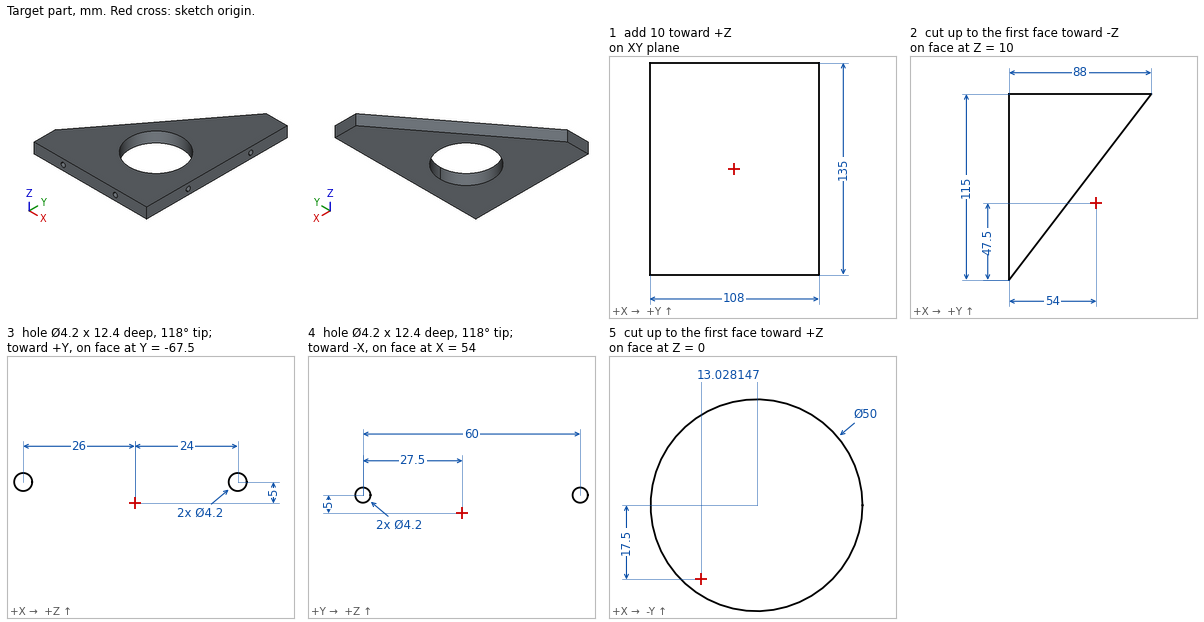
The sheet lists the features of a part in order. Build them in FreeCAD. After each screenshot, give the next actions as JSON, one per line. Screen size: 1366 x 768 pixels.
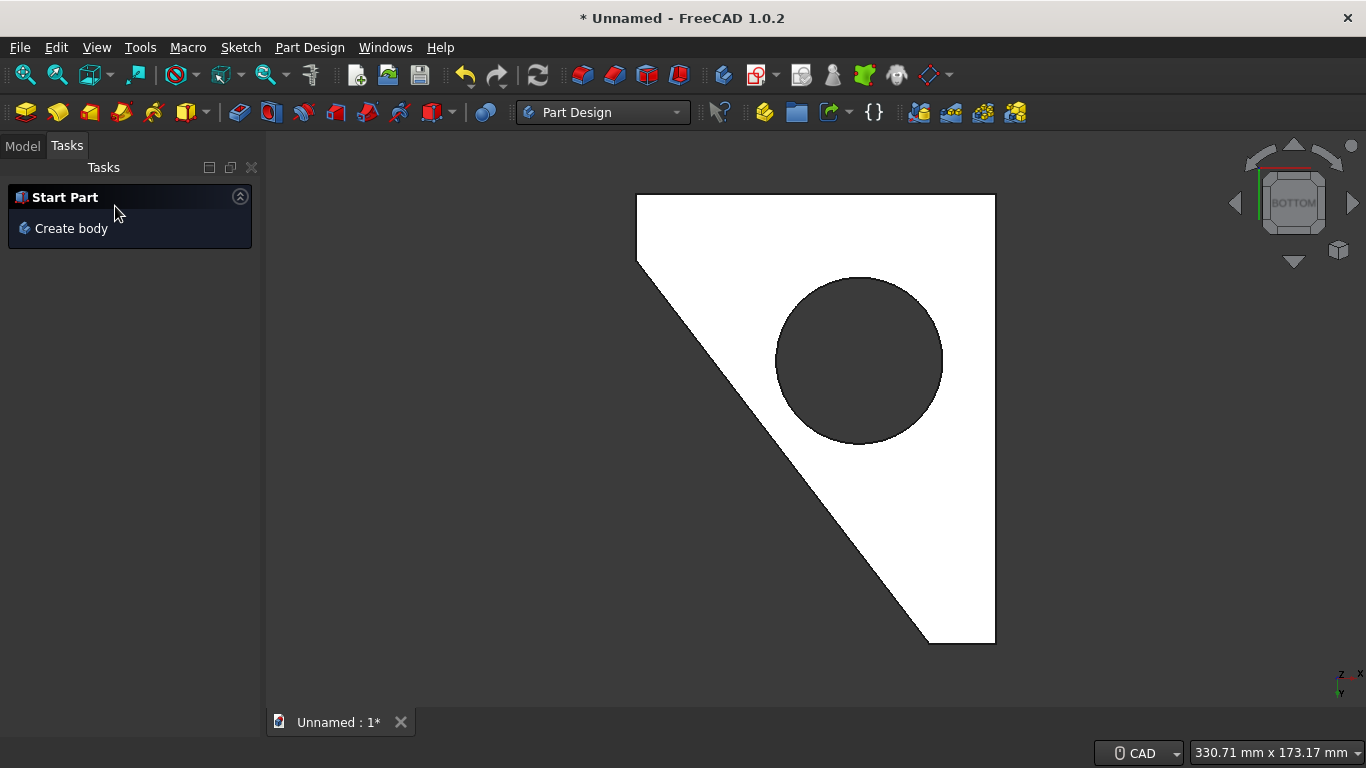
{"action": "key", "text": "0"}